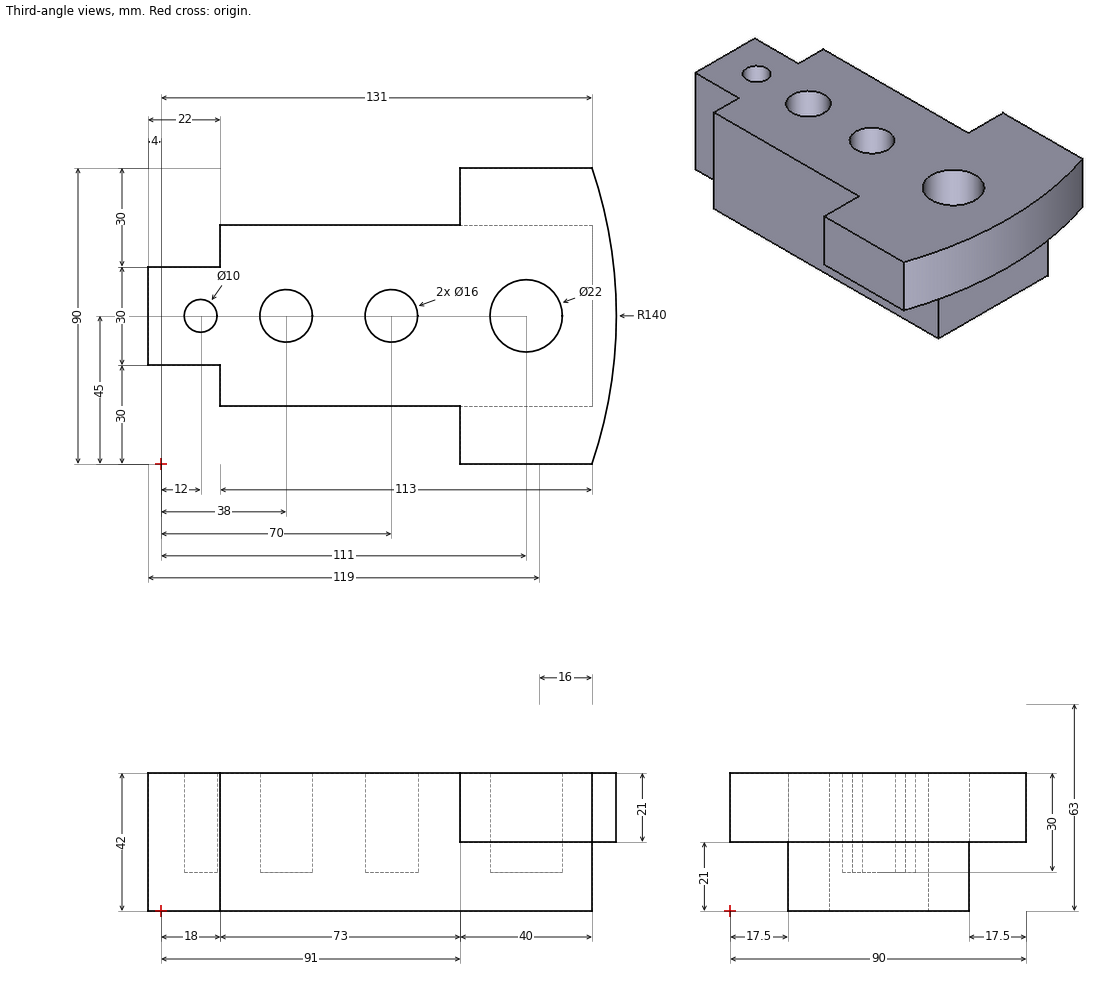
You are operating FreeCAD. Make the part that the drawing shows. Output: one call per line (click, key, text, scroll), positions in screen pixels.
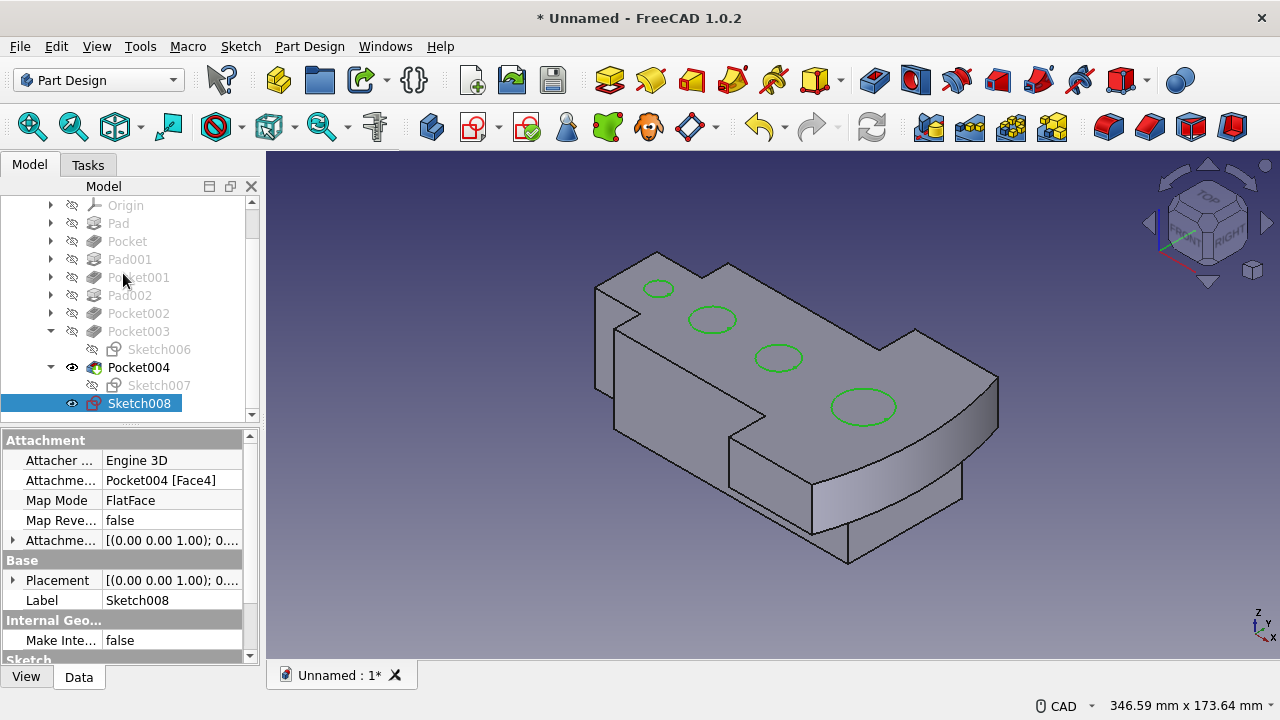
click(875, 80)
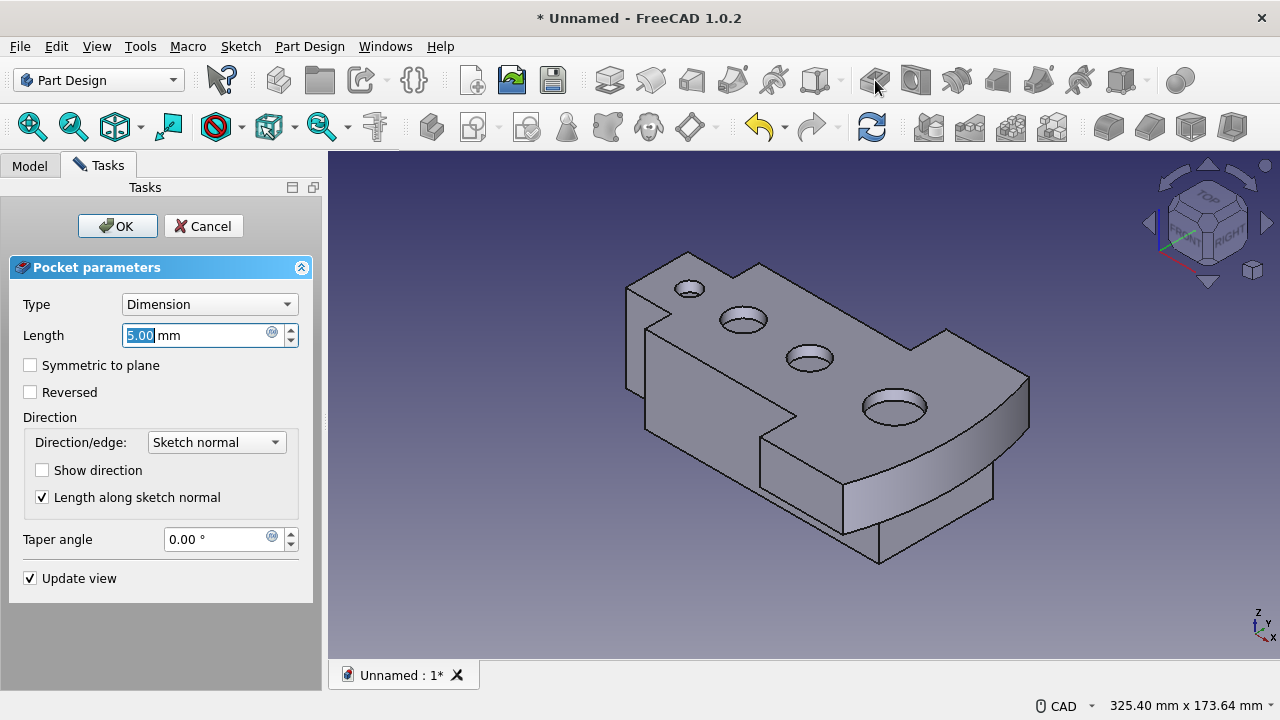
text(30)
key(Tab)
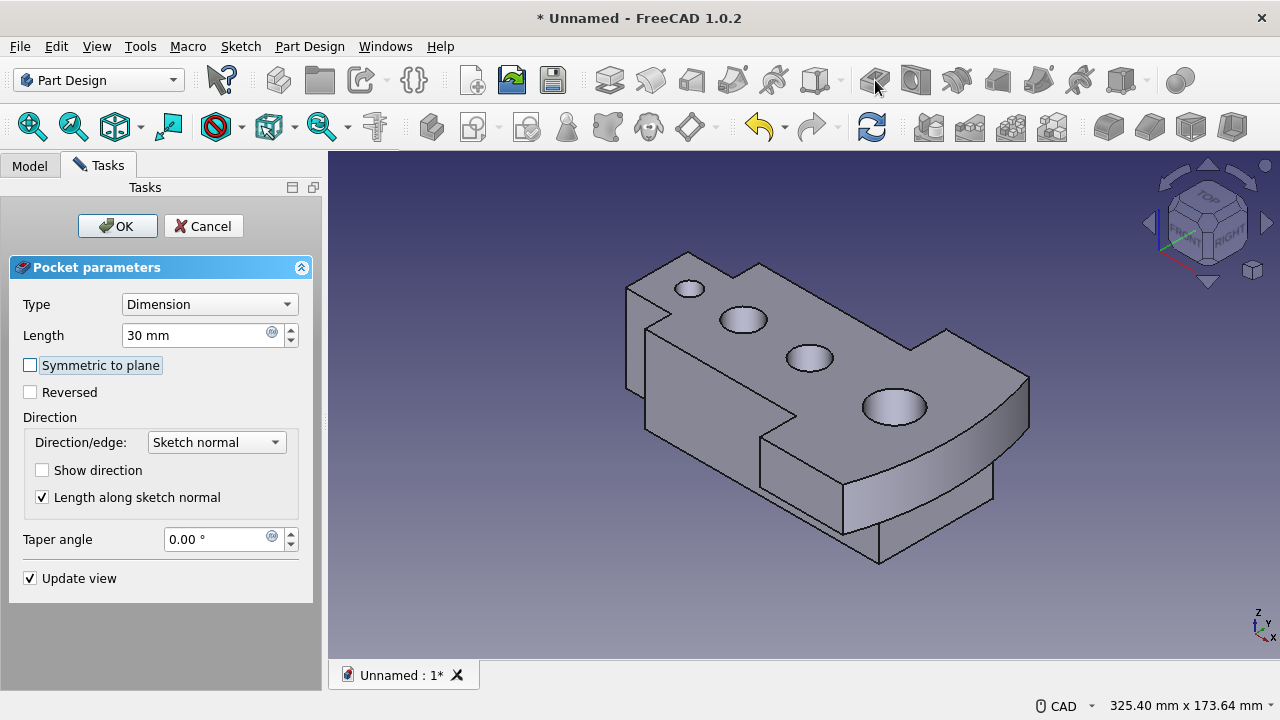
click(118, 226)